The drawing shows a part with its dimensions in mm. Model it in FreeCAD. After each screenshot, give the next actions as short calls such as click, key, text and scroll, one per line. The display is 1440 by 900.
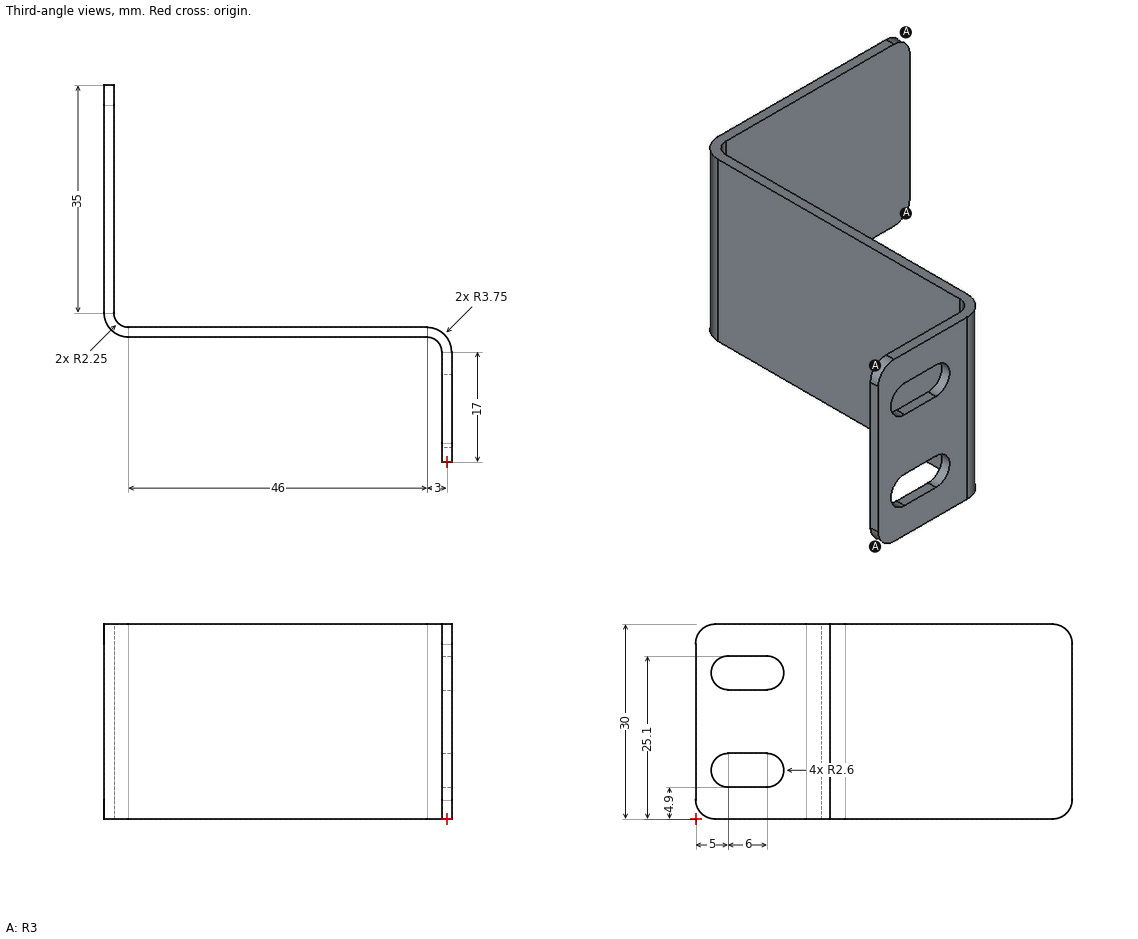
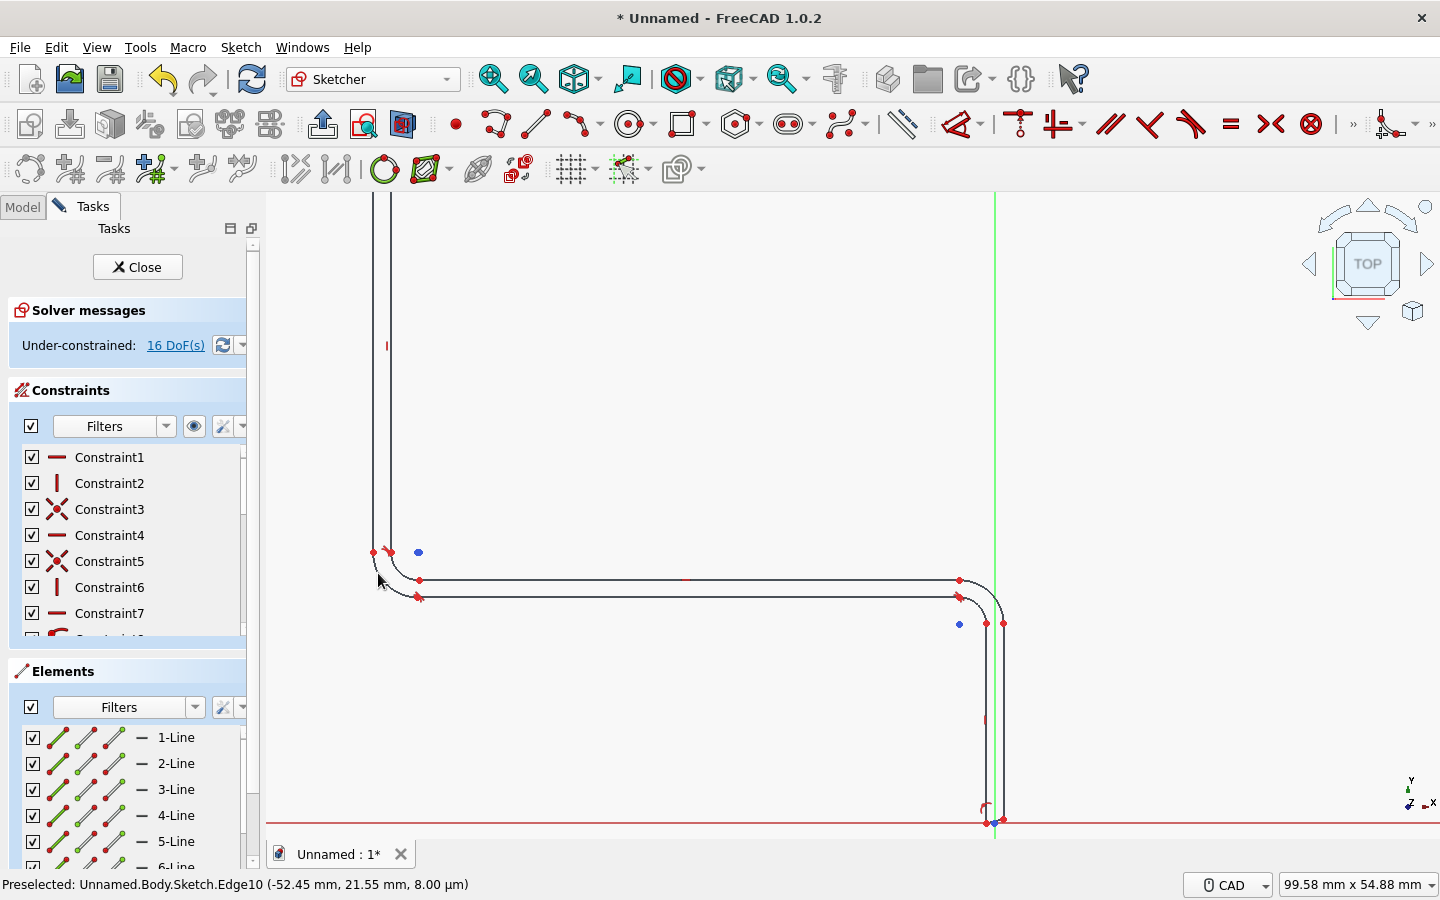
click(580, 597)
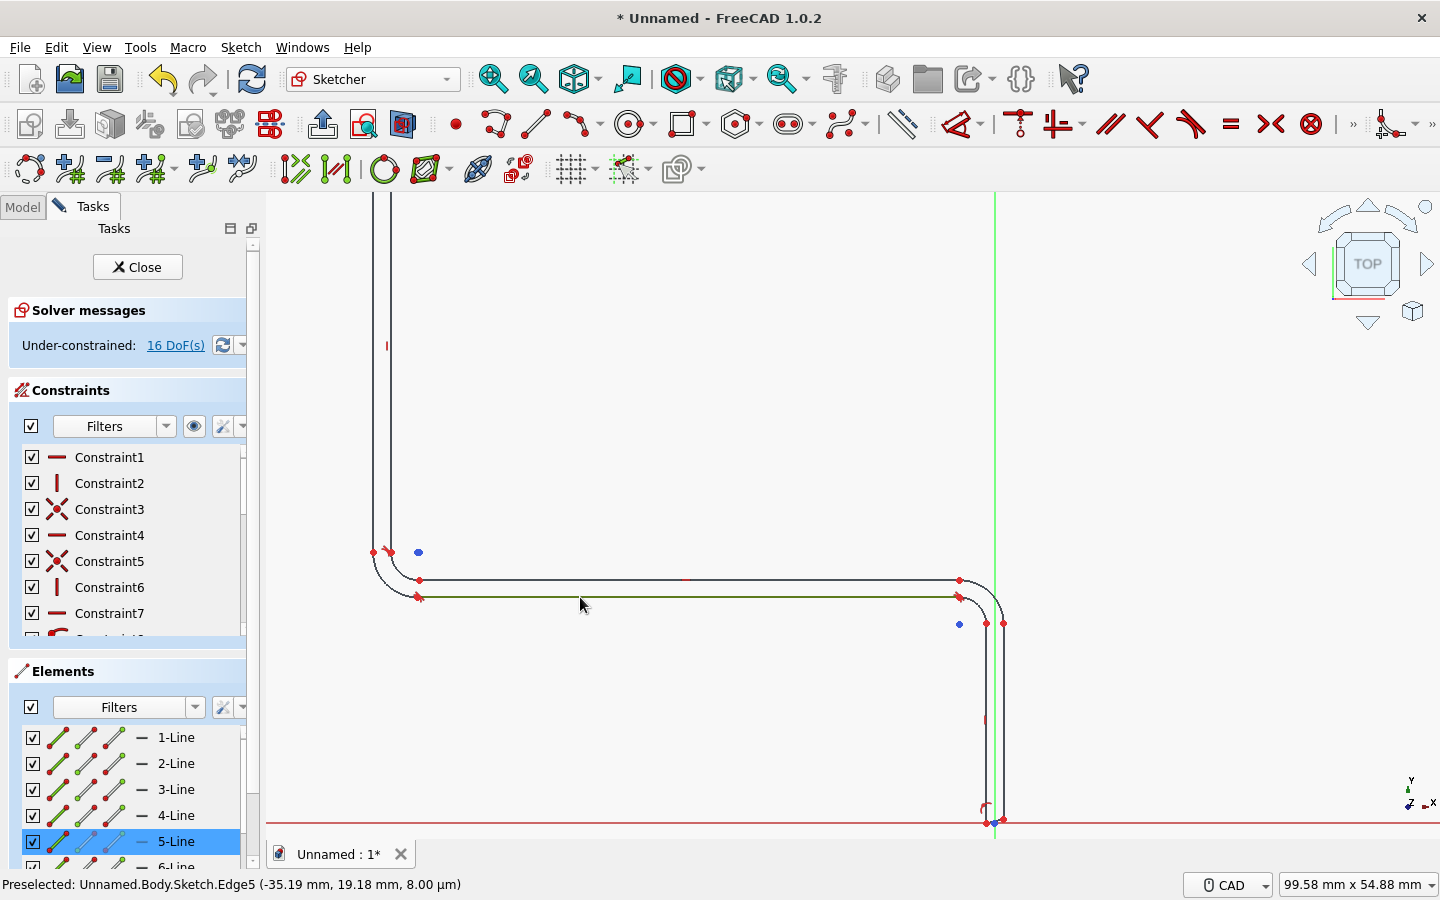
click(378, 573)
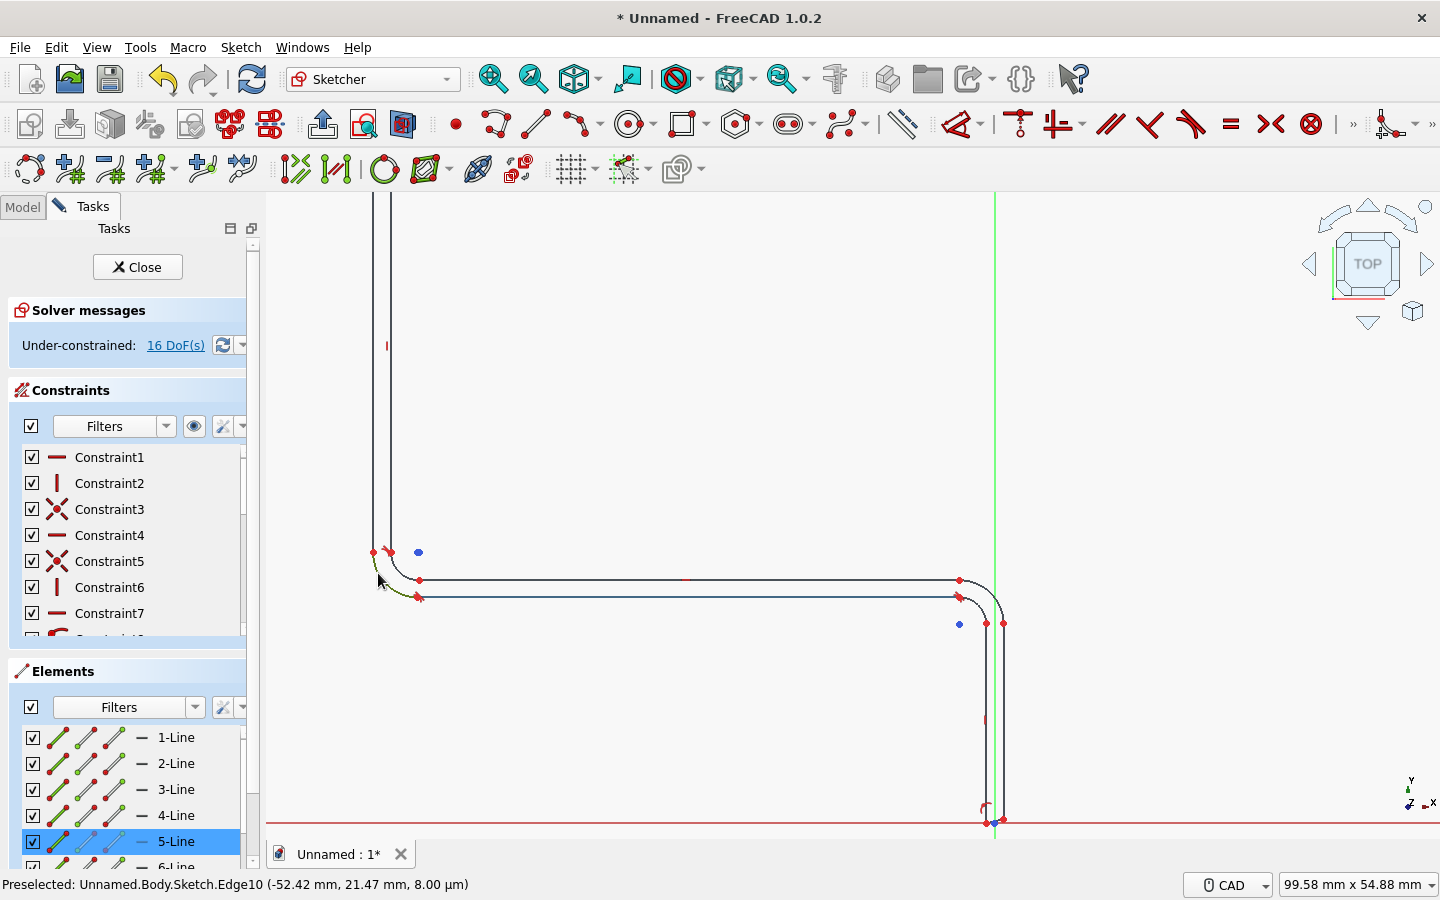
key(t)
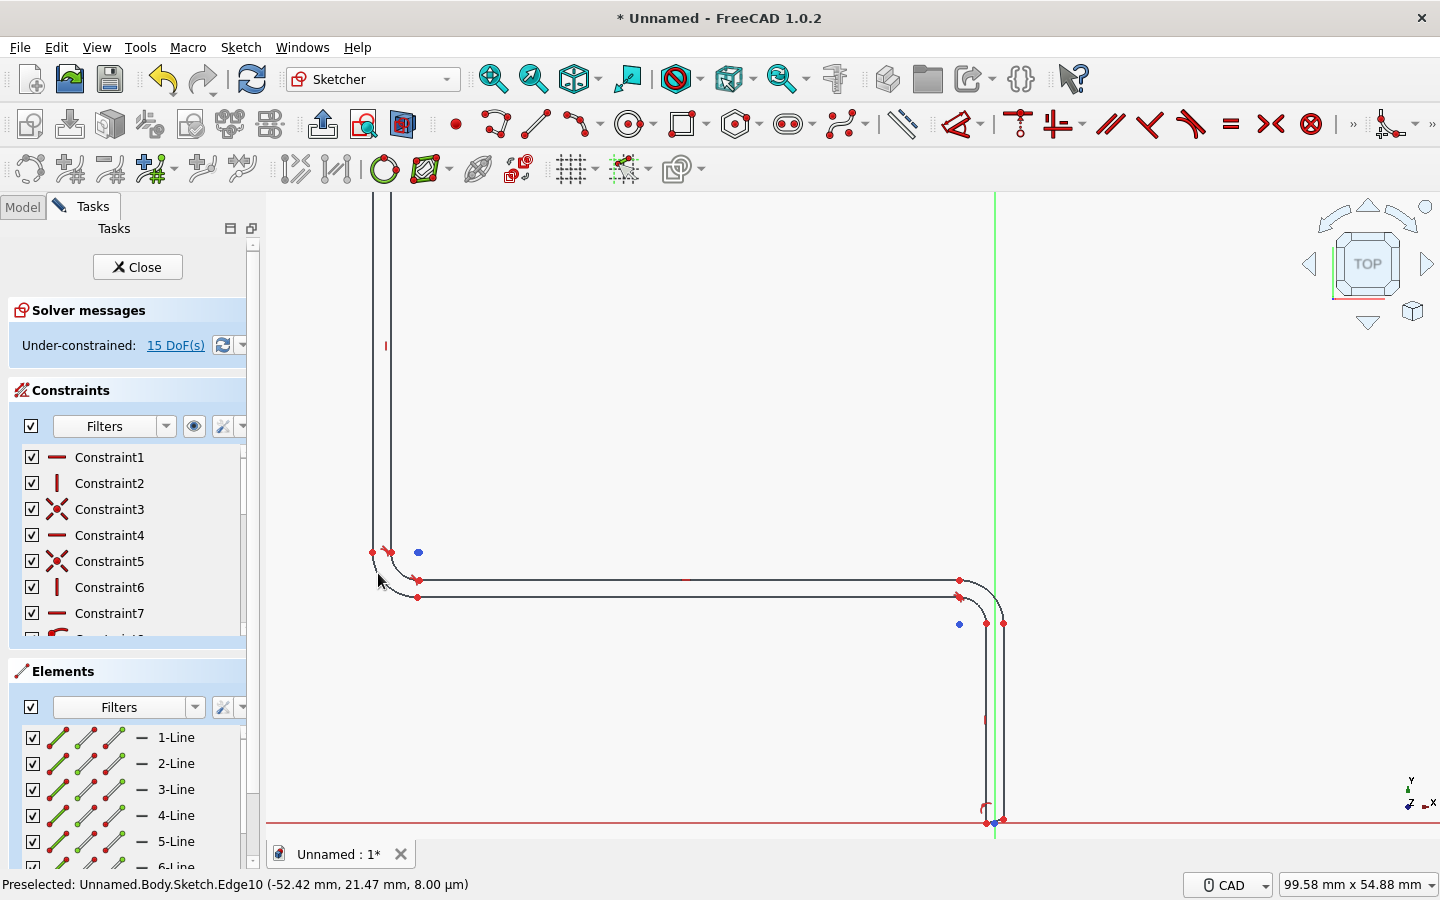
click(580, 597)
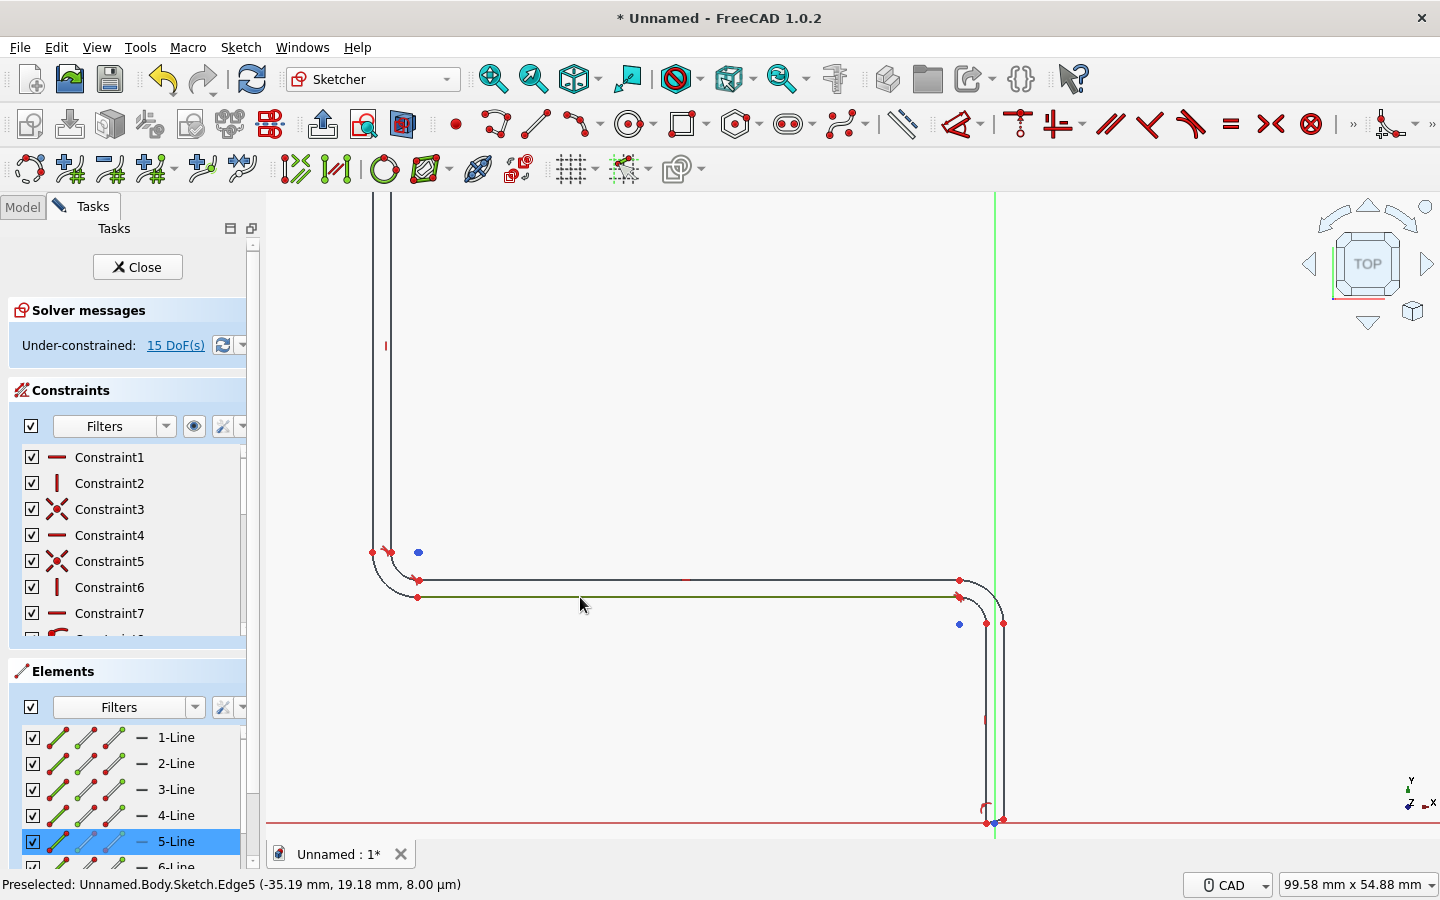
click(983, 612)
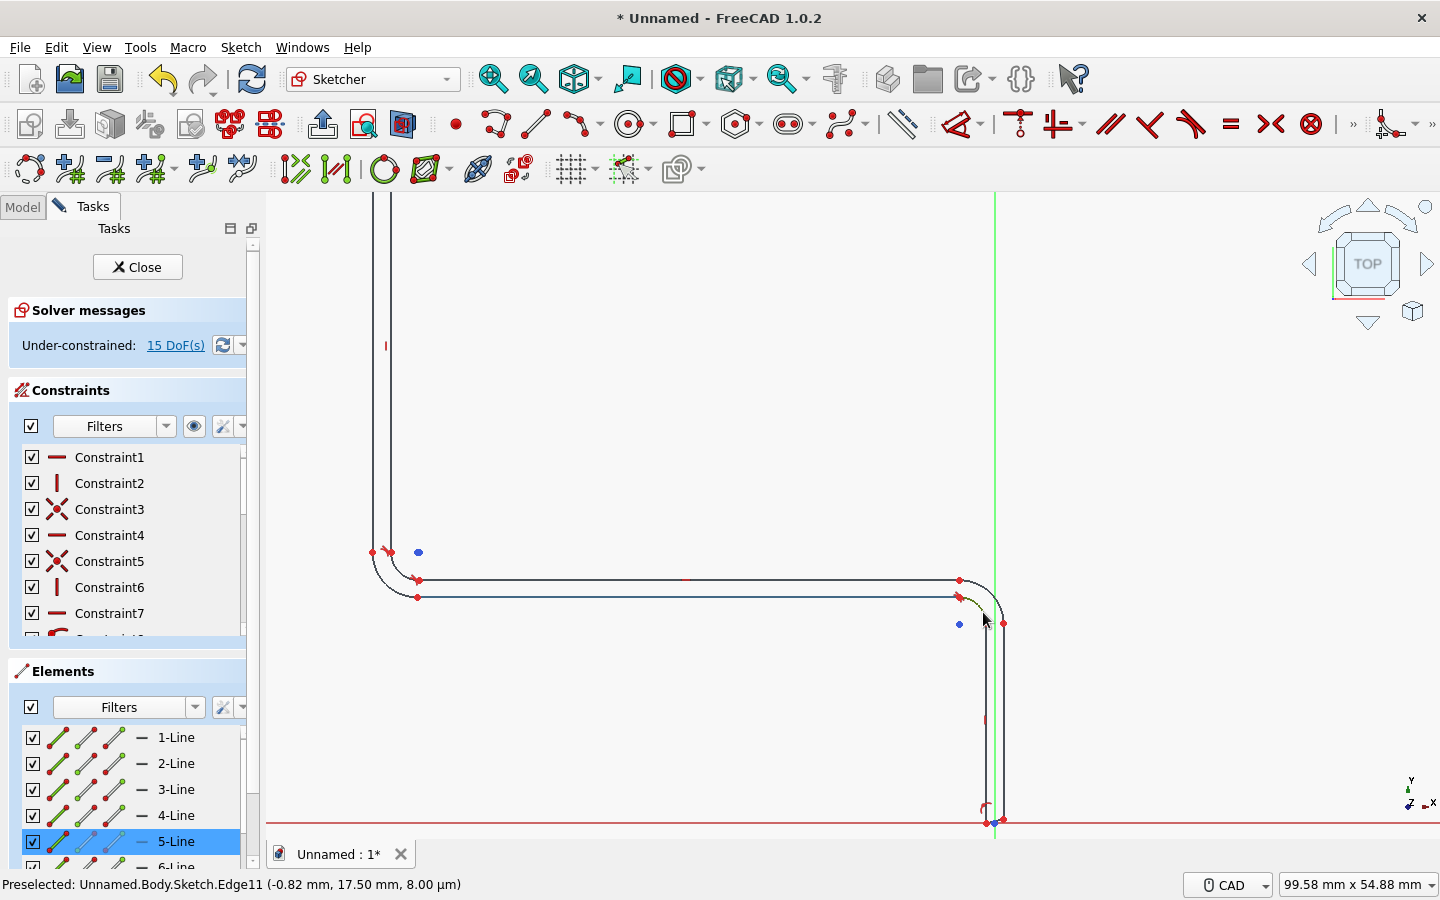
key(t)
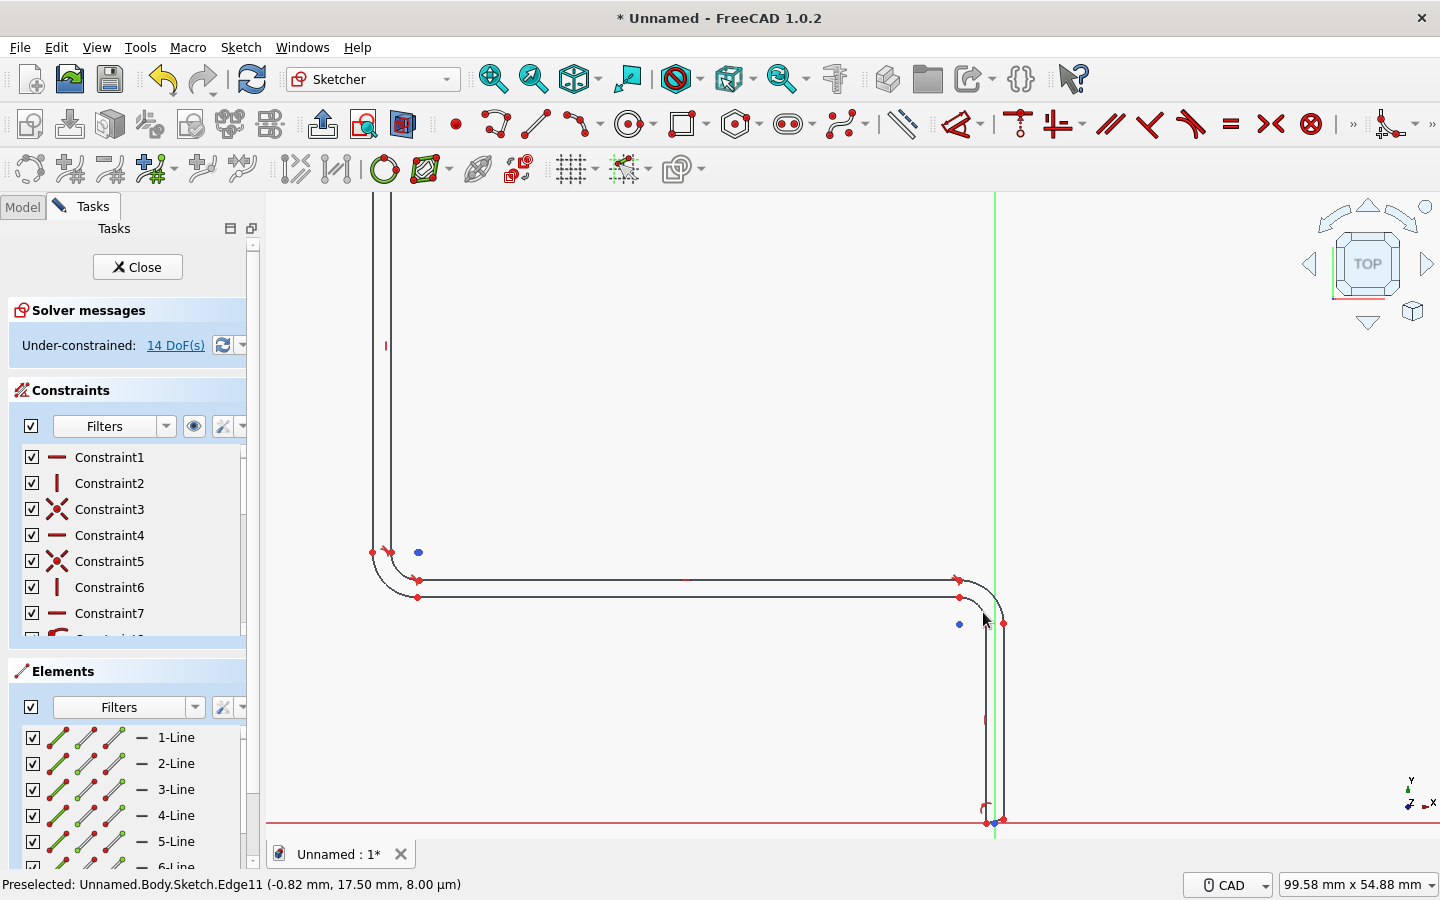
scroll(986, 684, up, 3)